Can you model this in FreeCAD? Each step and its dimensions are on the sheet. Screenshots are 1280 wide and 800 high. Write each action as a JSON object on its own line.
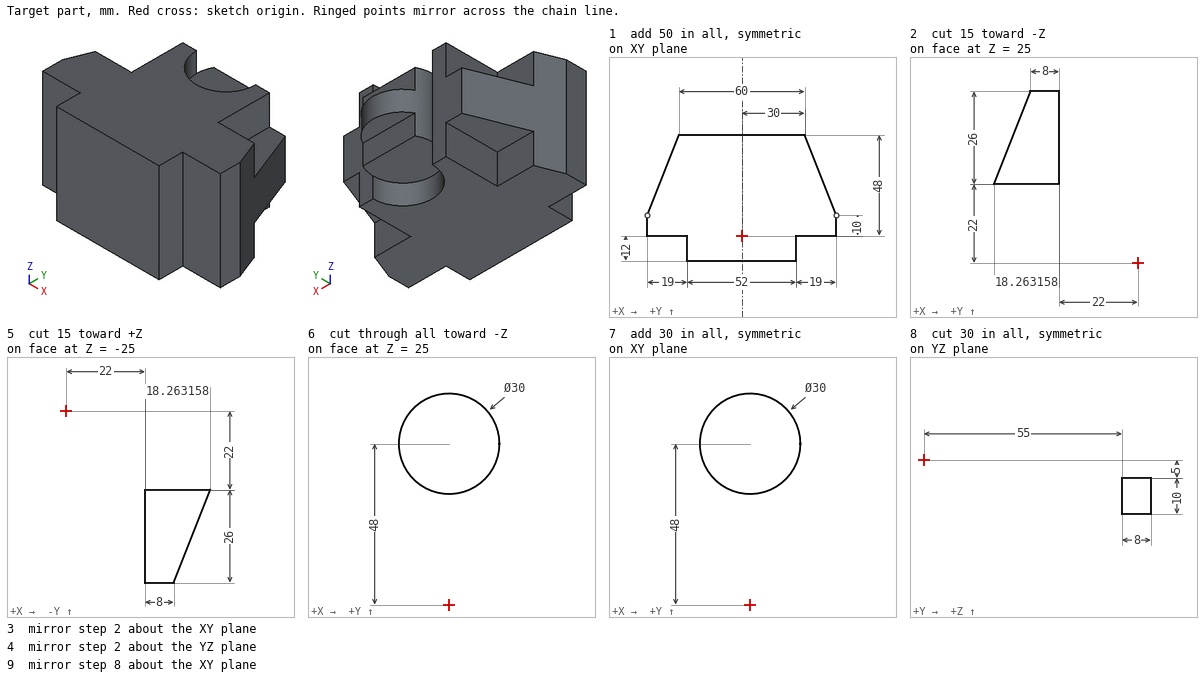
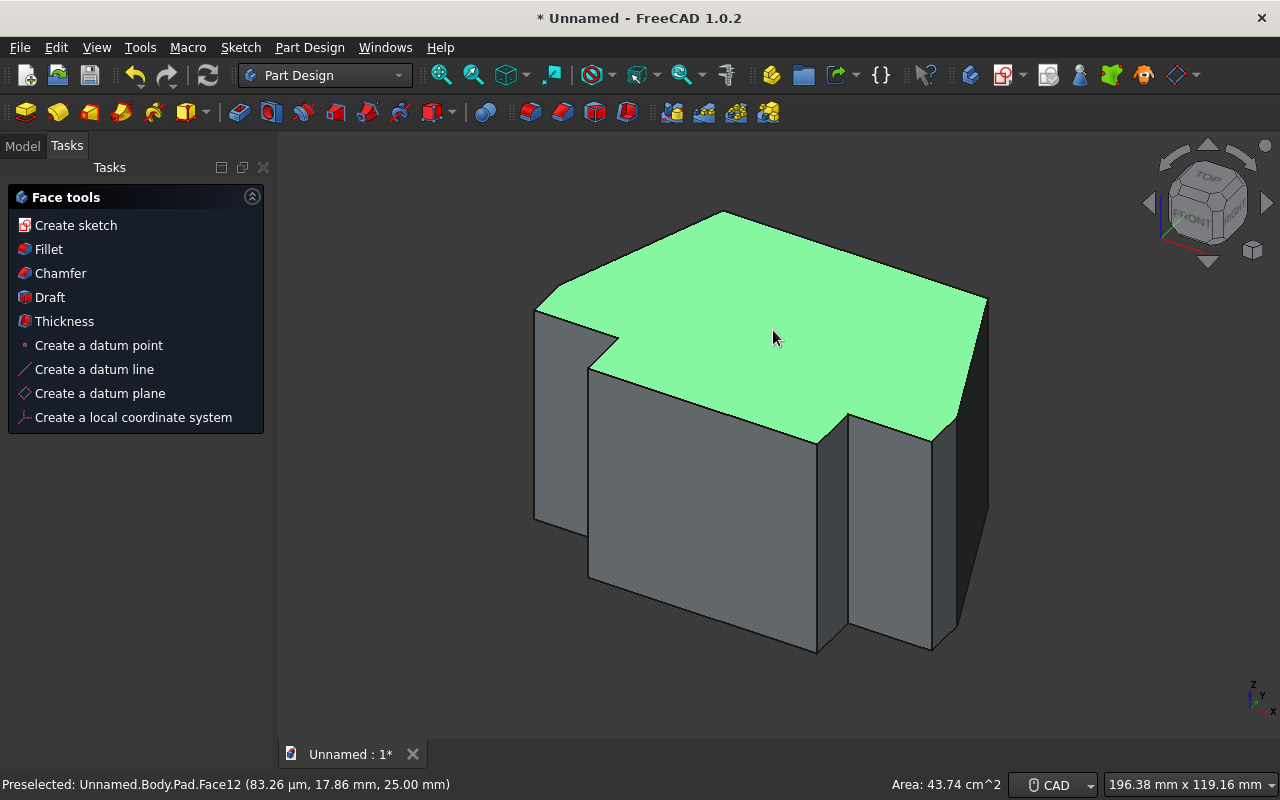
{"action": "left_click", "coordinate": [1004, 76]}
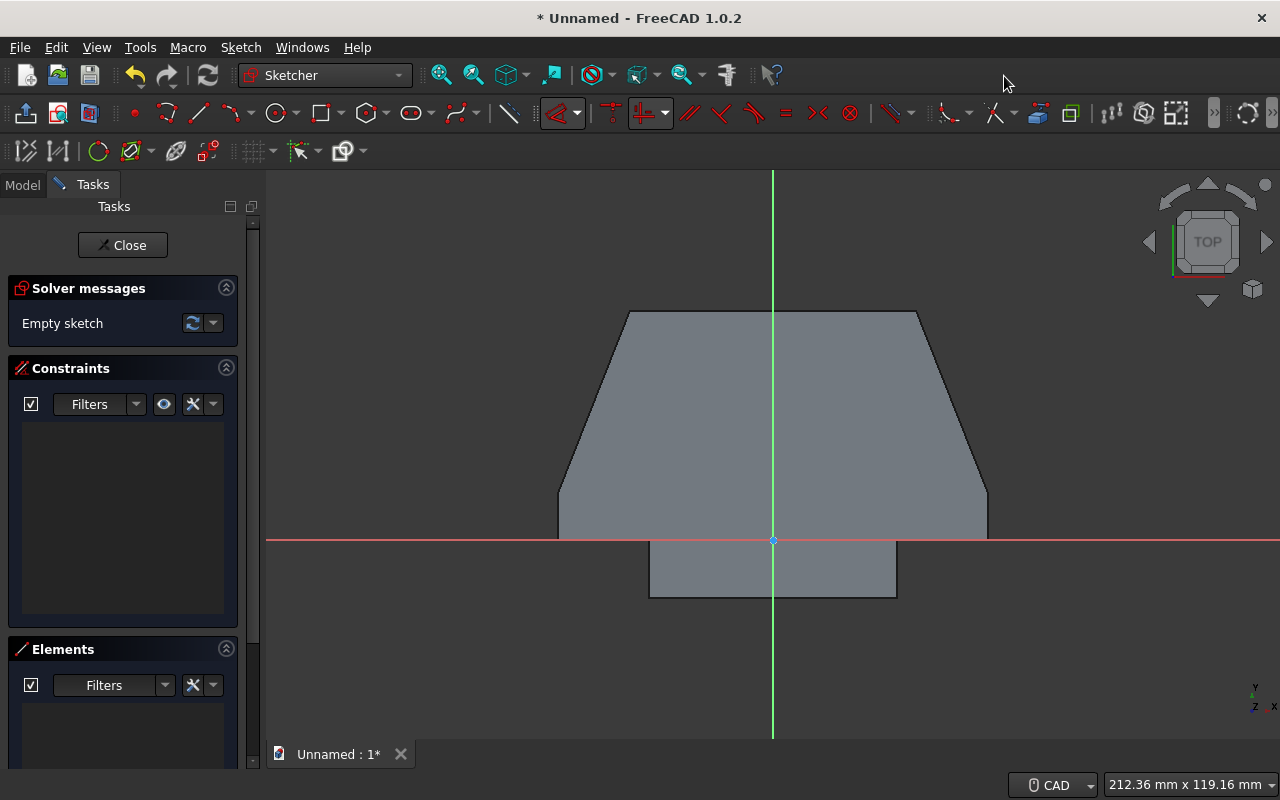
{"action": "scroll", "coordinate": [621, 368], "scroll_direction": "up", "scroll_amount": 2}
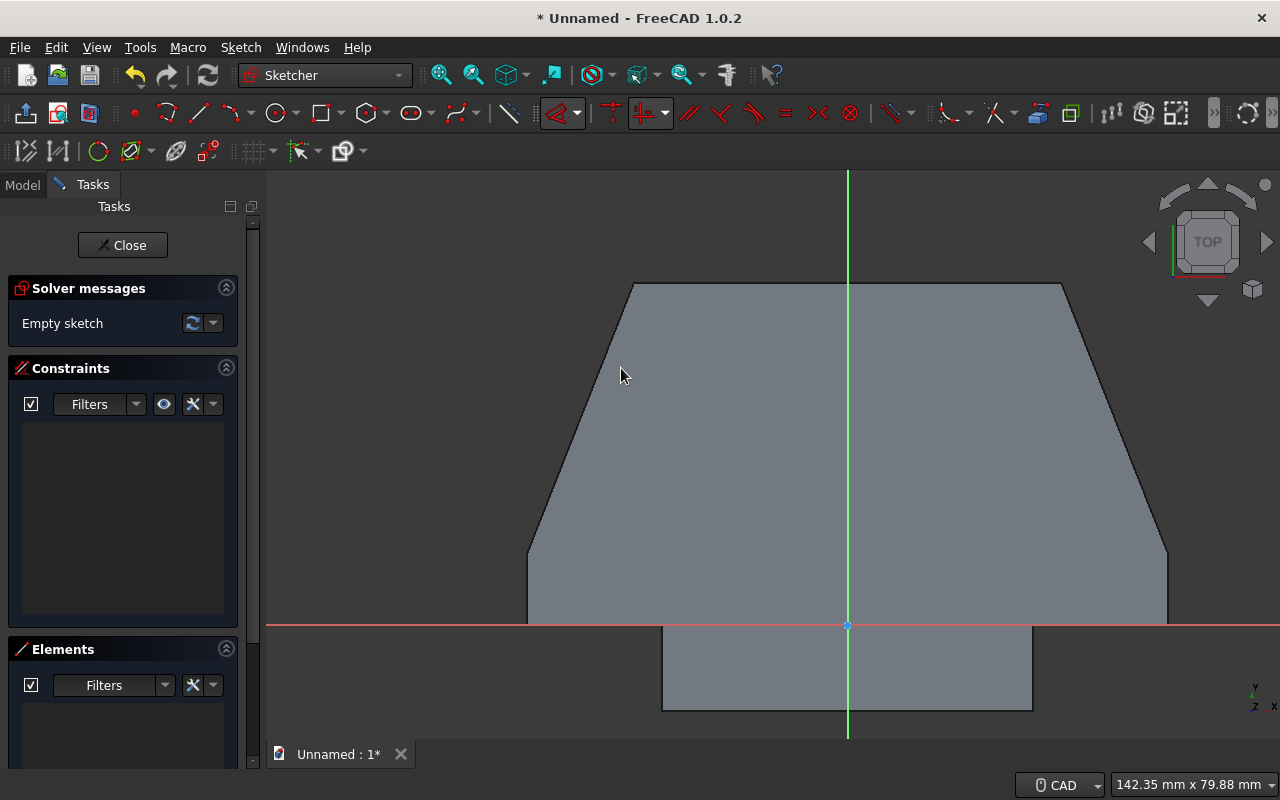
{"action": "left_click", "coordinate": [168, 114]}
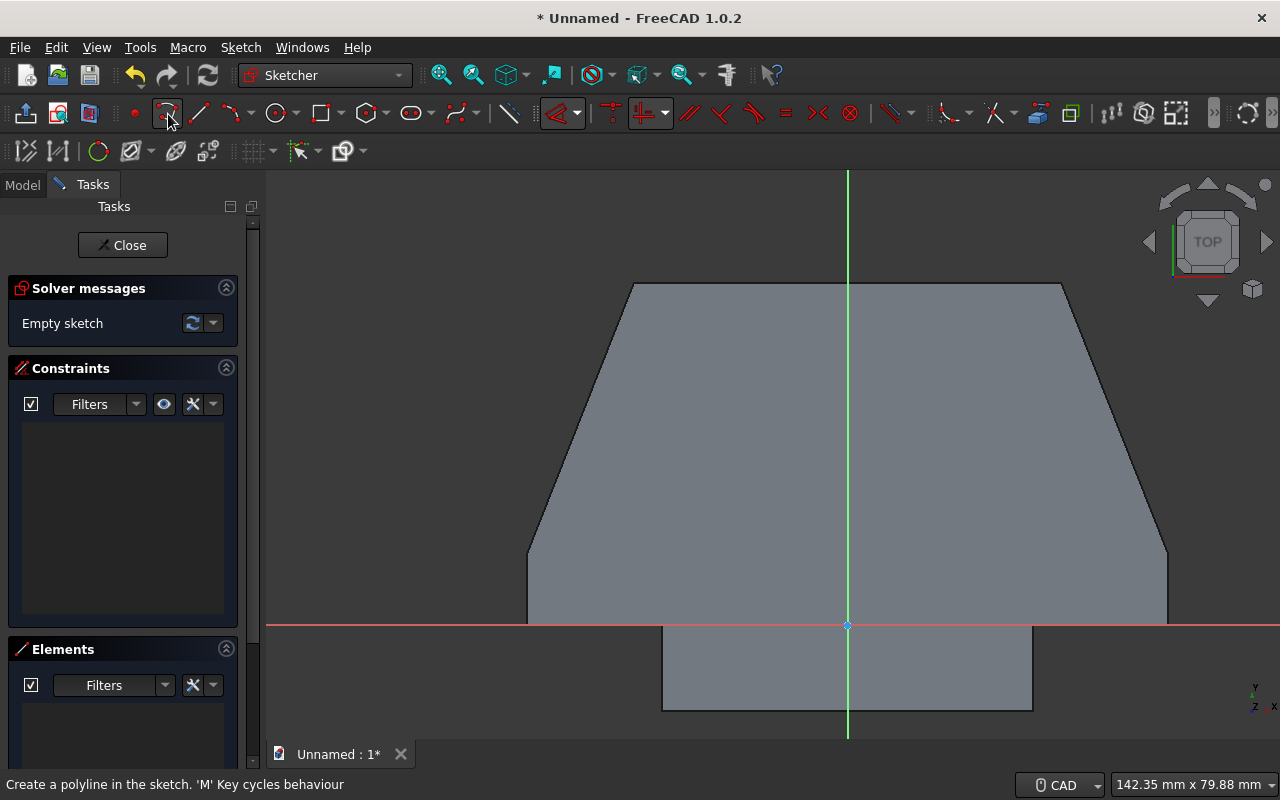
{"action": "left_click", "coordinate": [691, 468]}
{"action": "left_click", "coordinate": [691, 283]}
{"action": "left_click", "coordinate": [634, 283]}
{"action": "left_click", "coordinate": [561, 468]}
{"action": "left_click", "coordinate": [691, 469]}
{"action": "key", "text": "Escape"}
{"action": "key", "text": "Escape"}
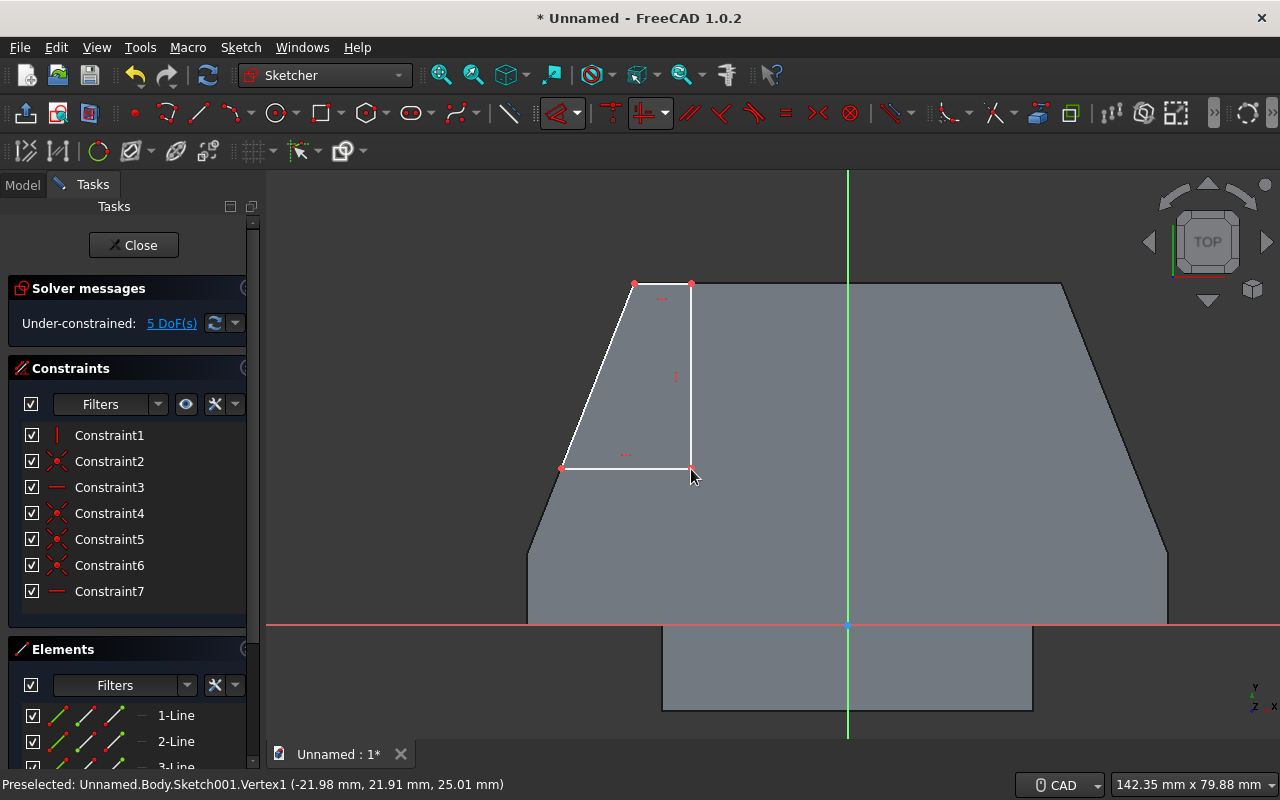
{"action": "left_click", "coordinate": [674, 284]}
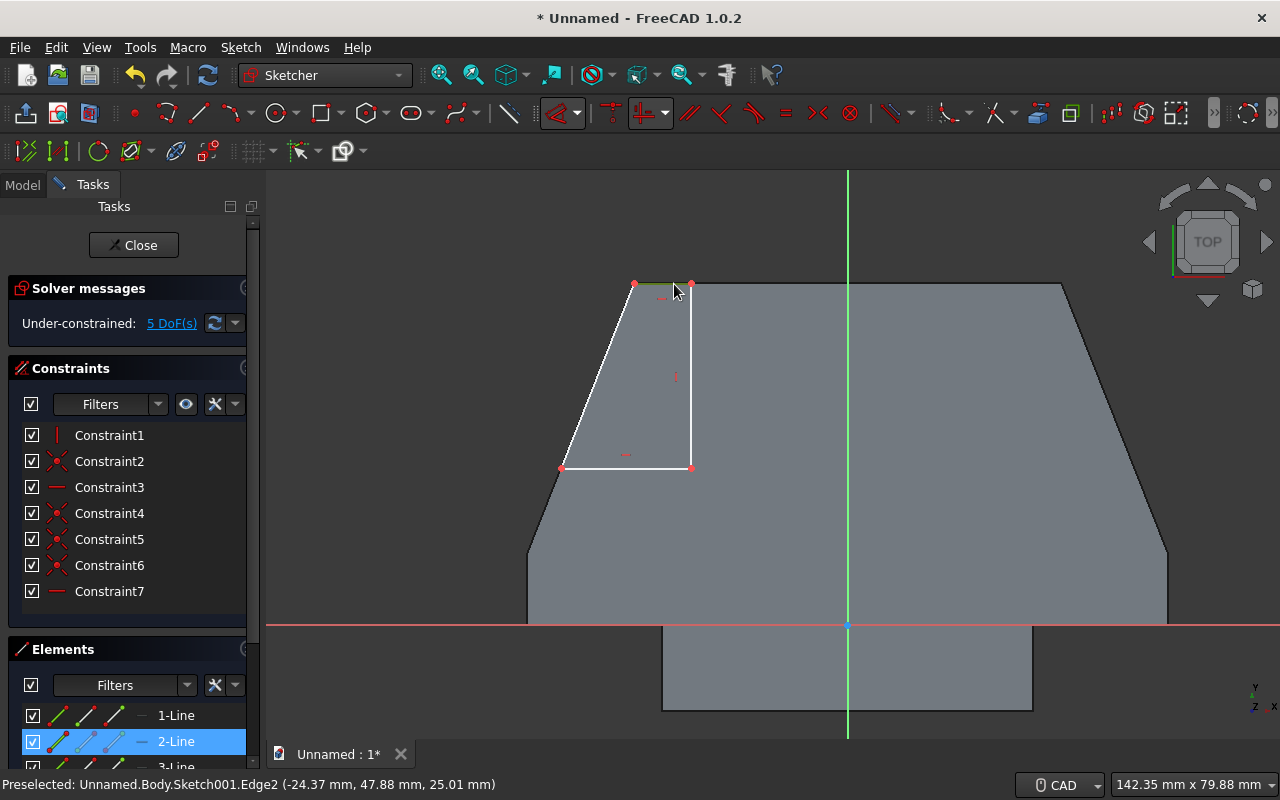
{"action": "left_click", "coordinate": [580, 114]}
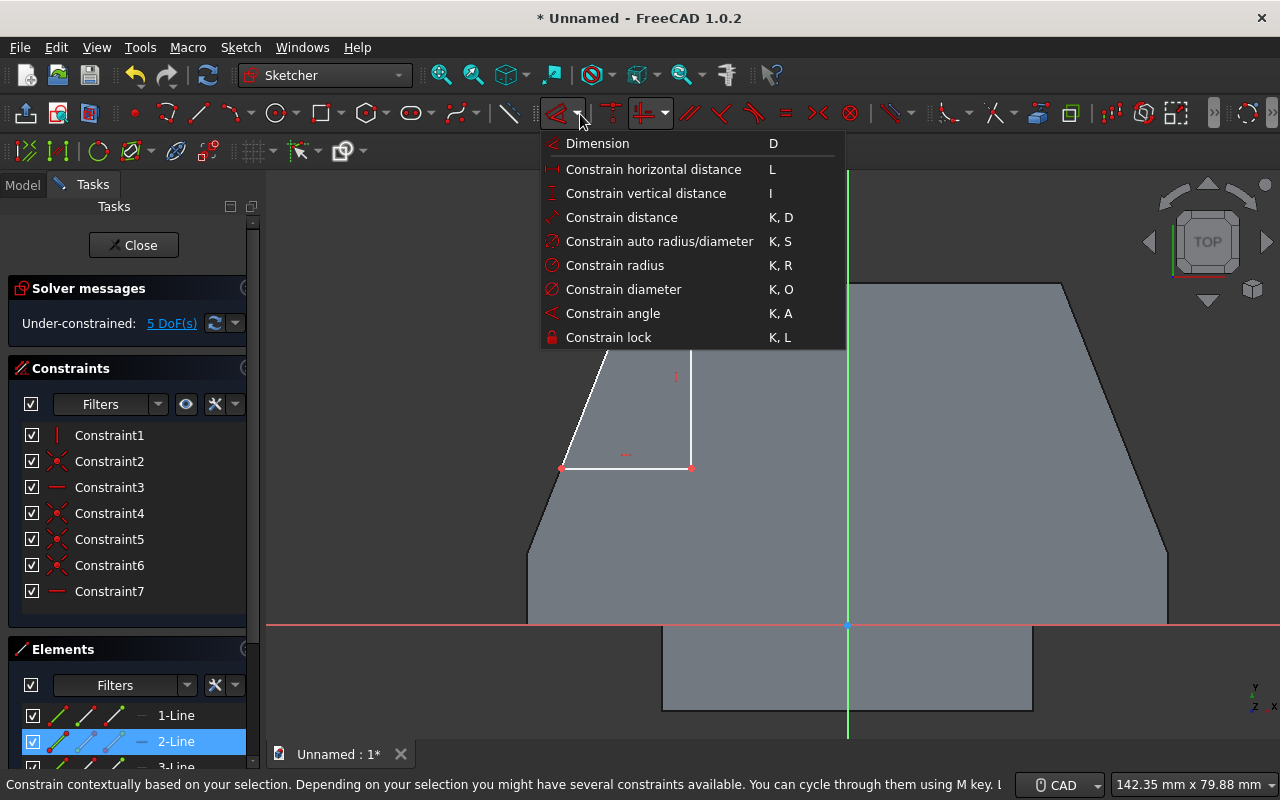
{"action": "left_click", "coordinate": [693, 169]}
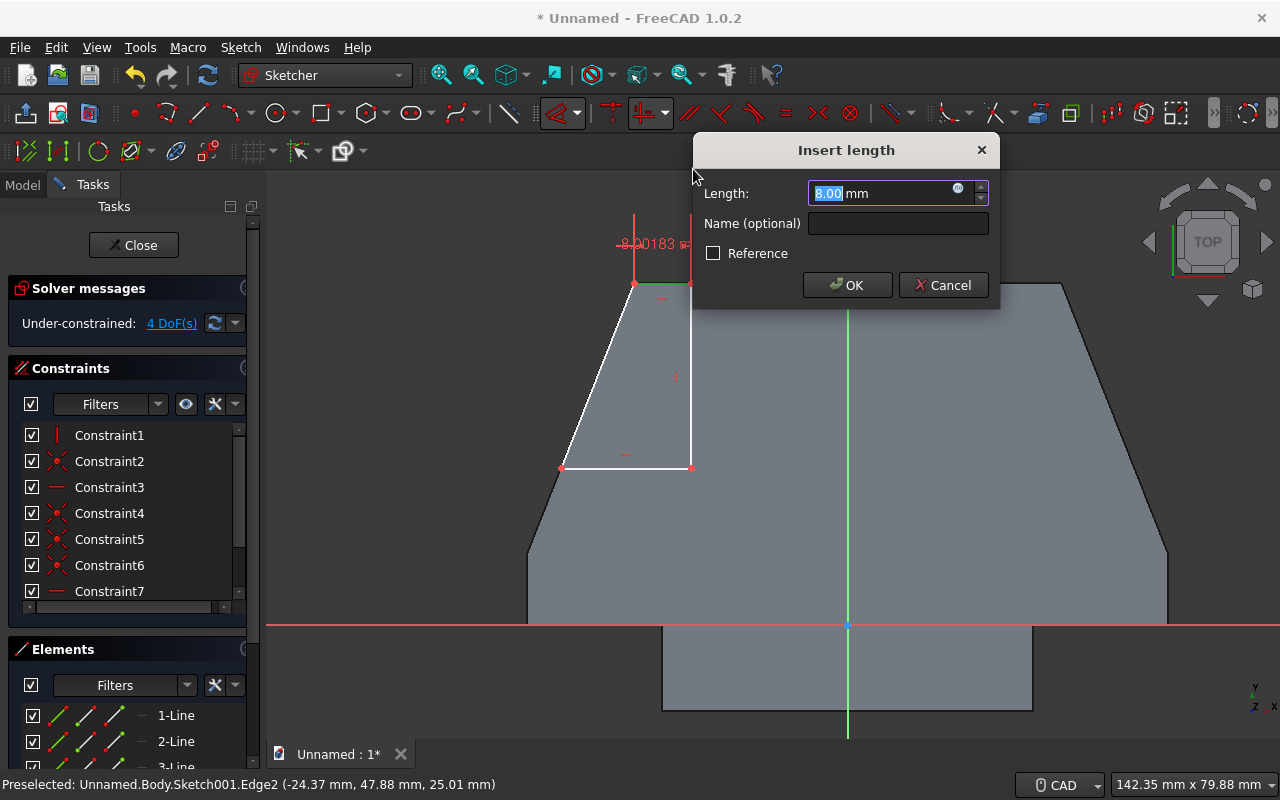
{"action": "type", "text": "8"}
{"action": "key", "text": "Return"}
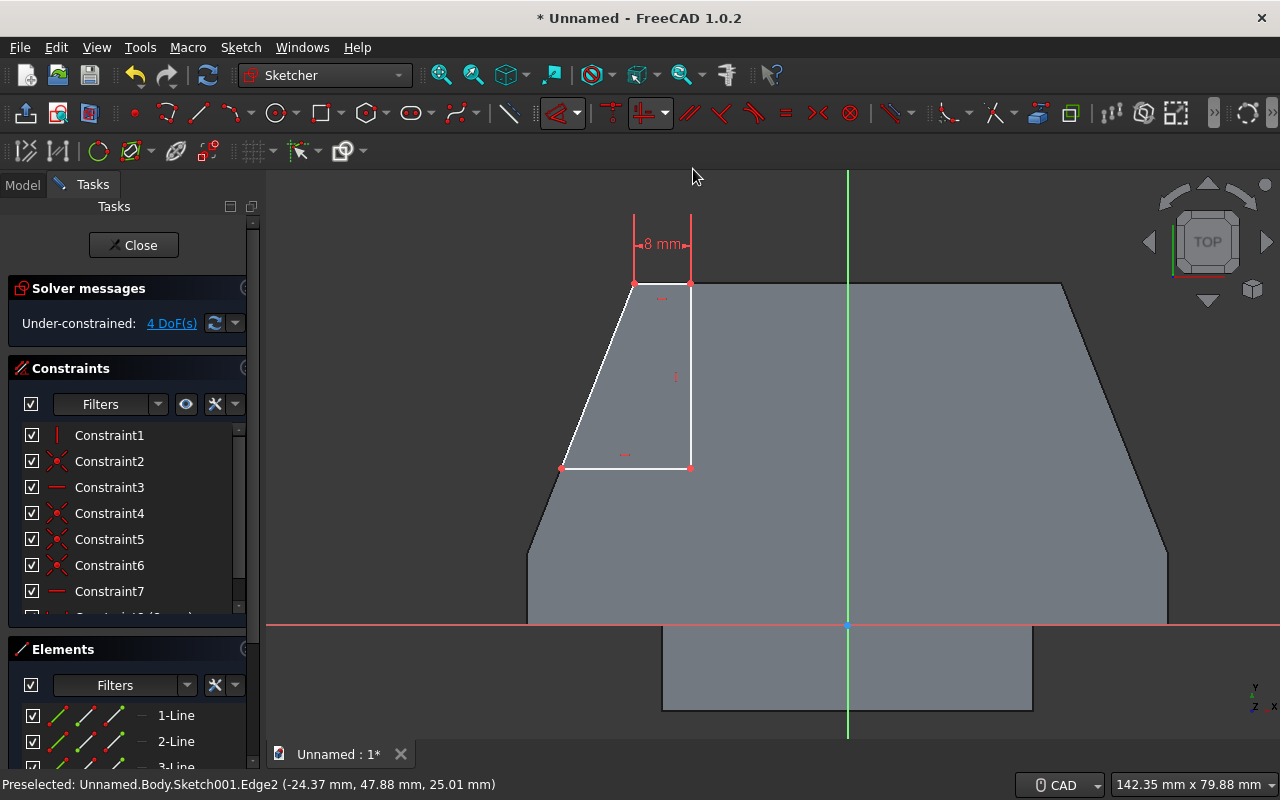
{"action": "left_click", "coordinate": [691, 414]}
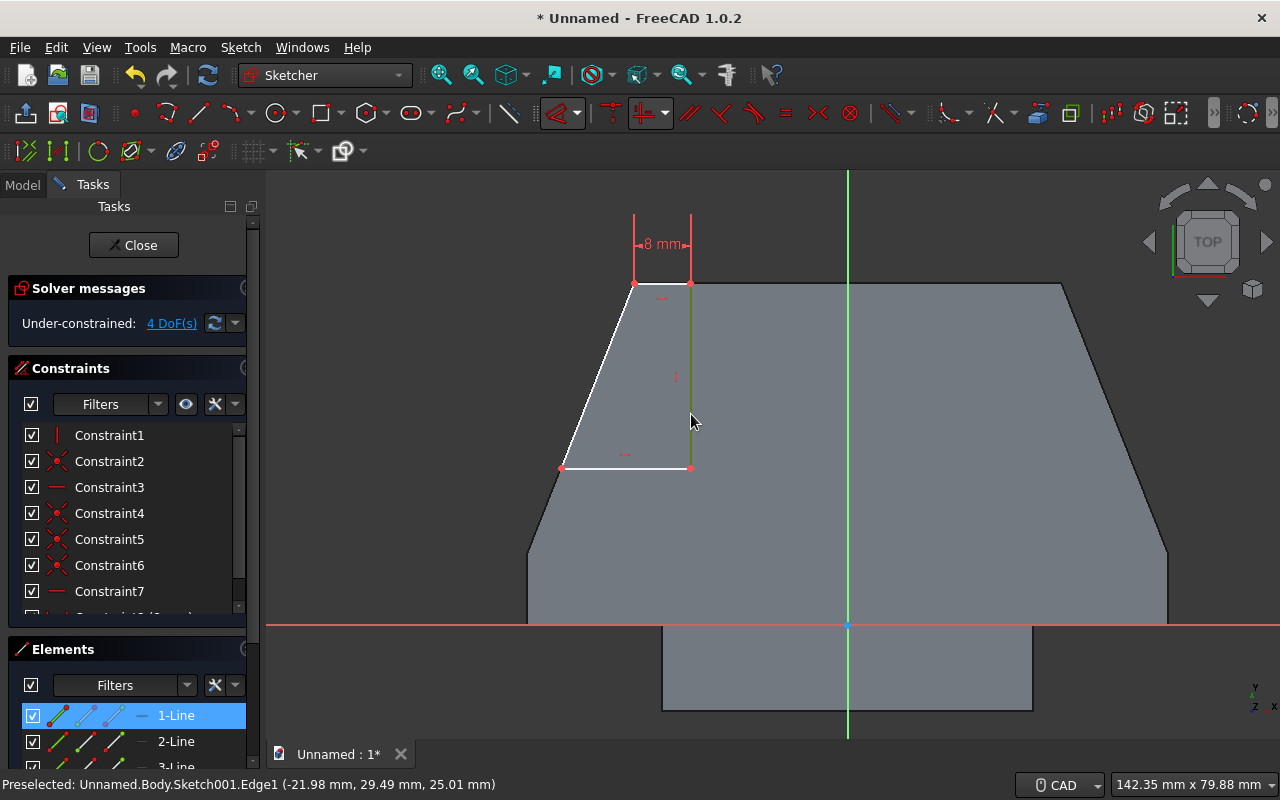
{"action": "key", "text": "i"}